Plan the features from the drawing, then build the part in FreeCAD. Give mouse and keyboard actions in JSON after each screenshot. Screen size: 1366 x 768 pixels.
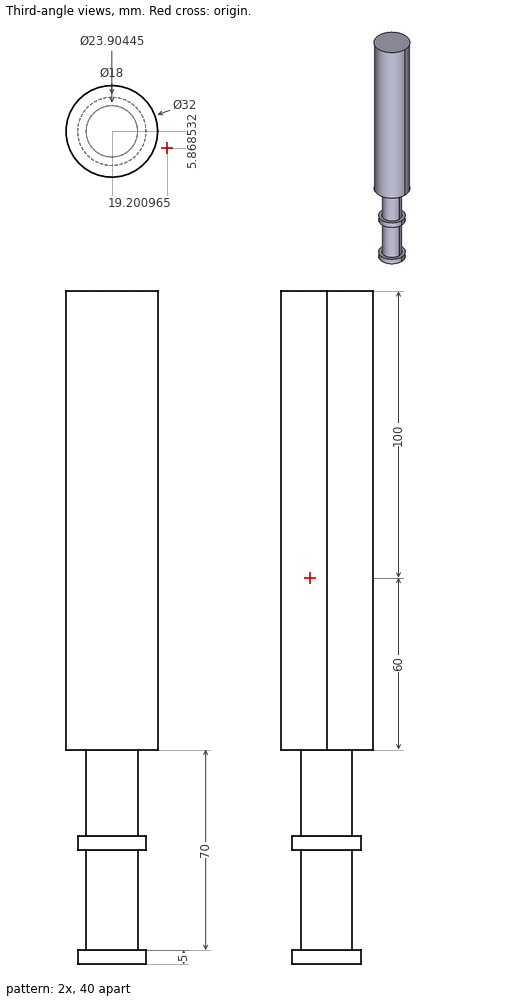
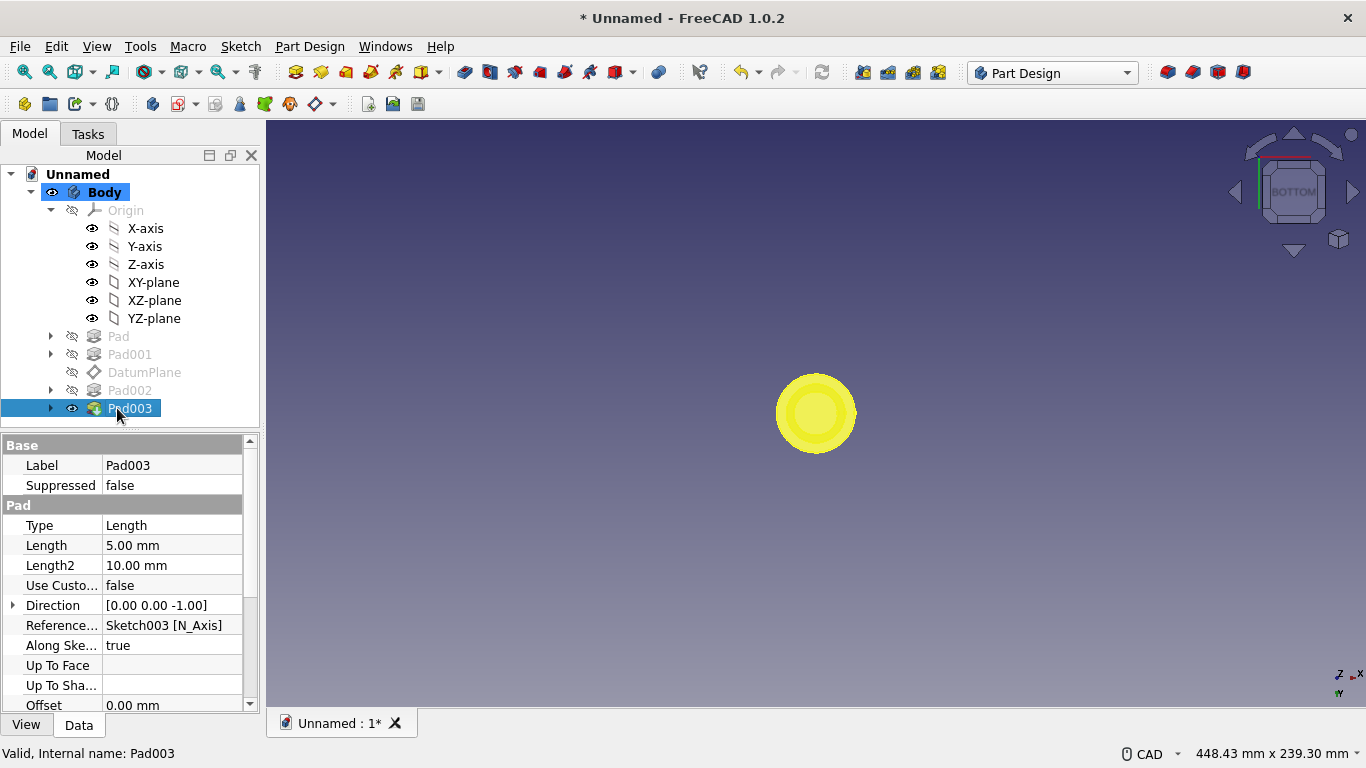
{"action": "left_click", "coordinate": [888, 72]}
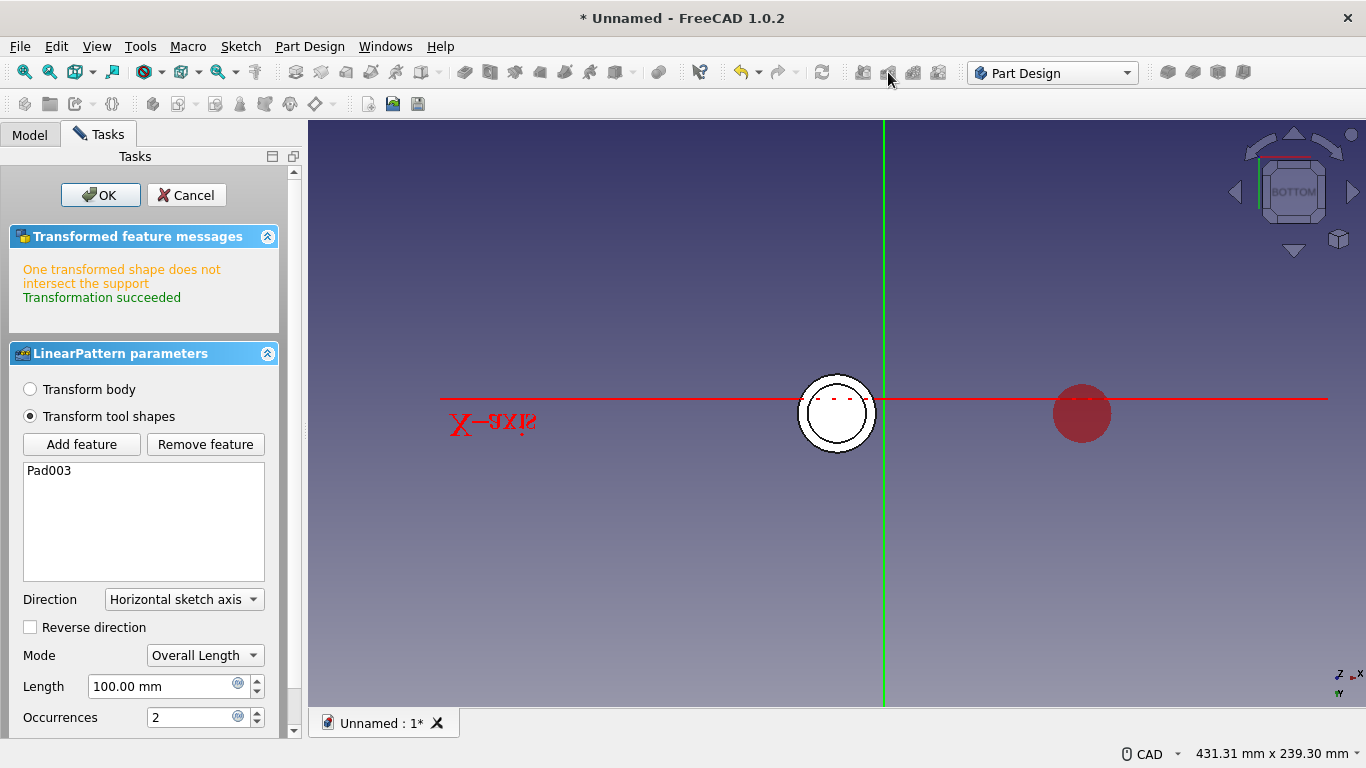
{"action": "left_click", "coordinate": [185, 600]}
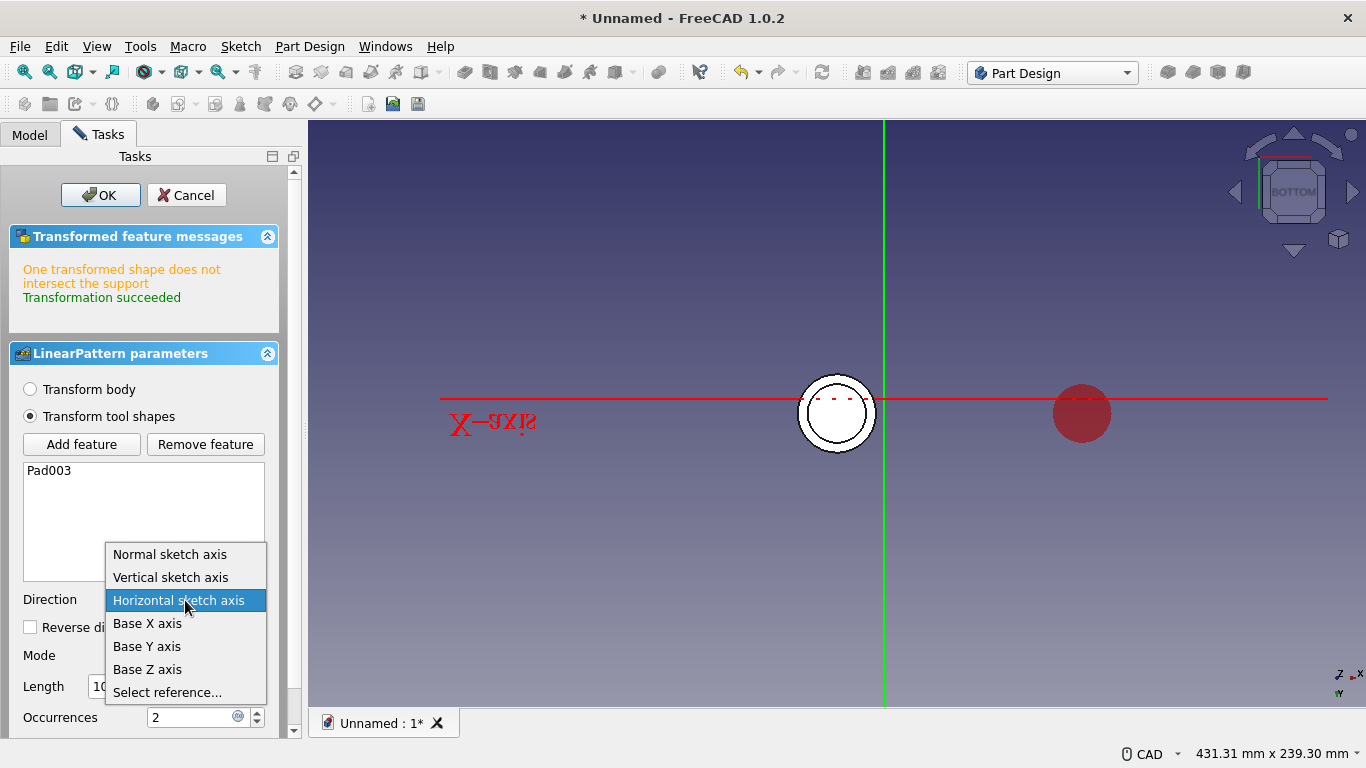
{"action": "left_click", "coordinate": [184, 670]}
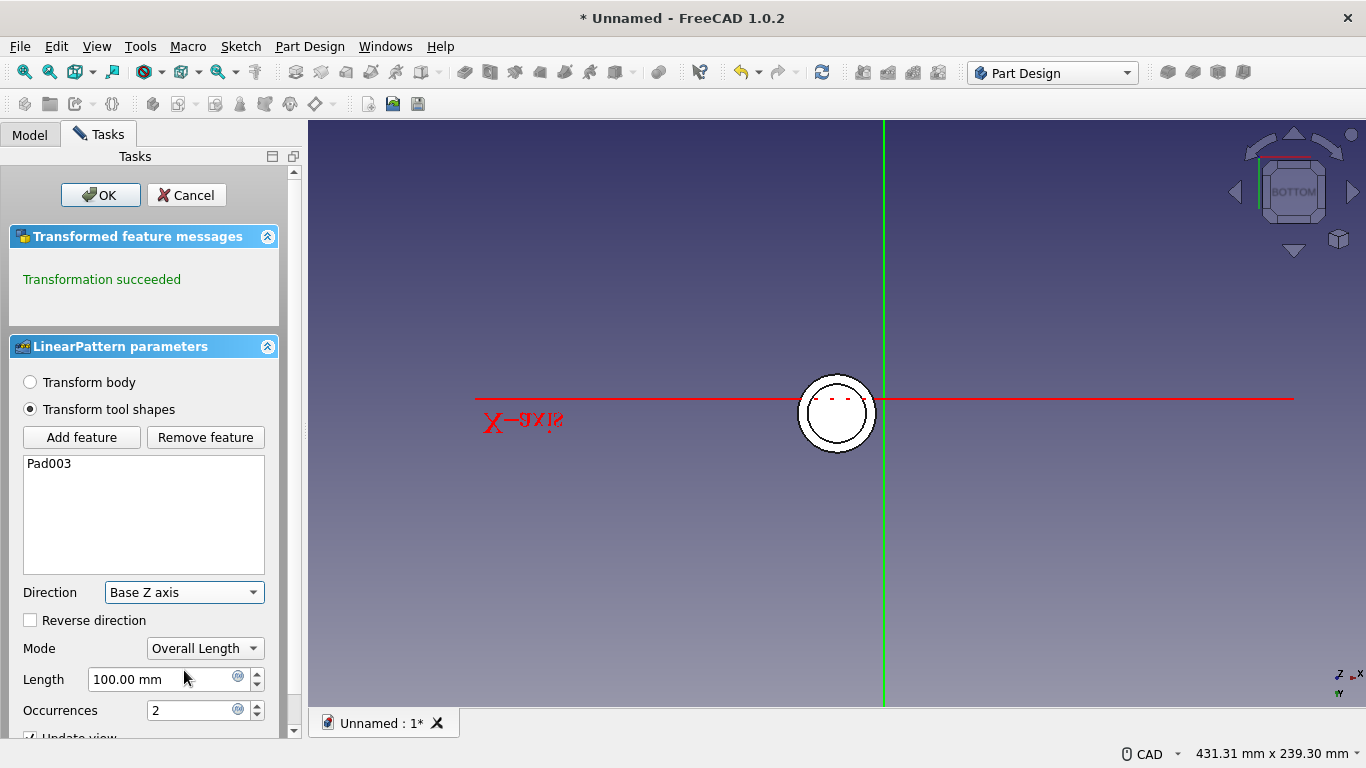
{"action": "left_click", "coordinate": [206, 648]}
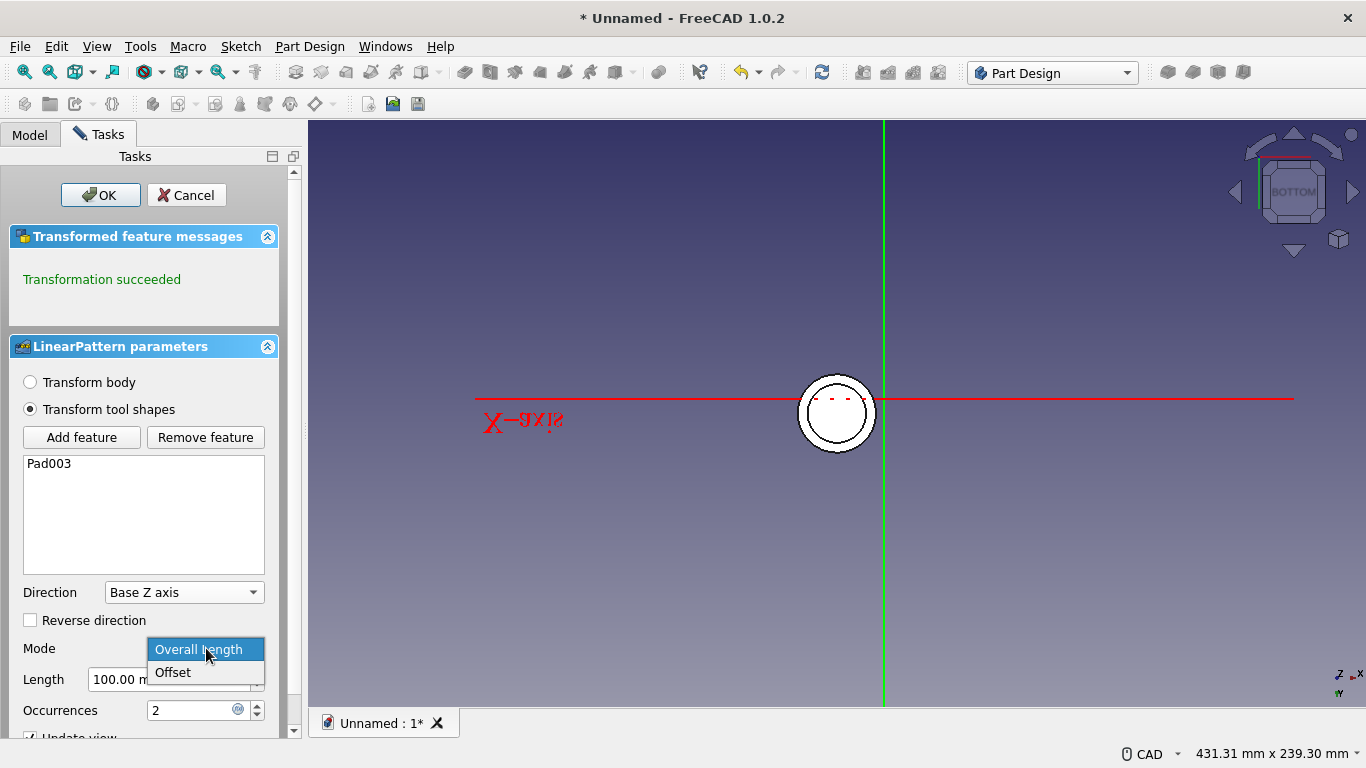
{"action": "left_click", "coordinate": [204, 672]}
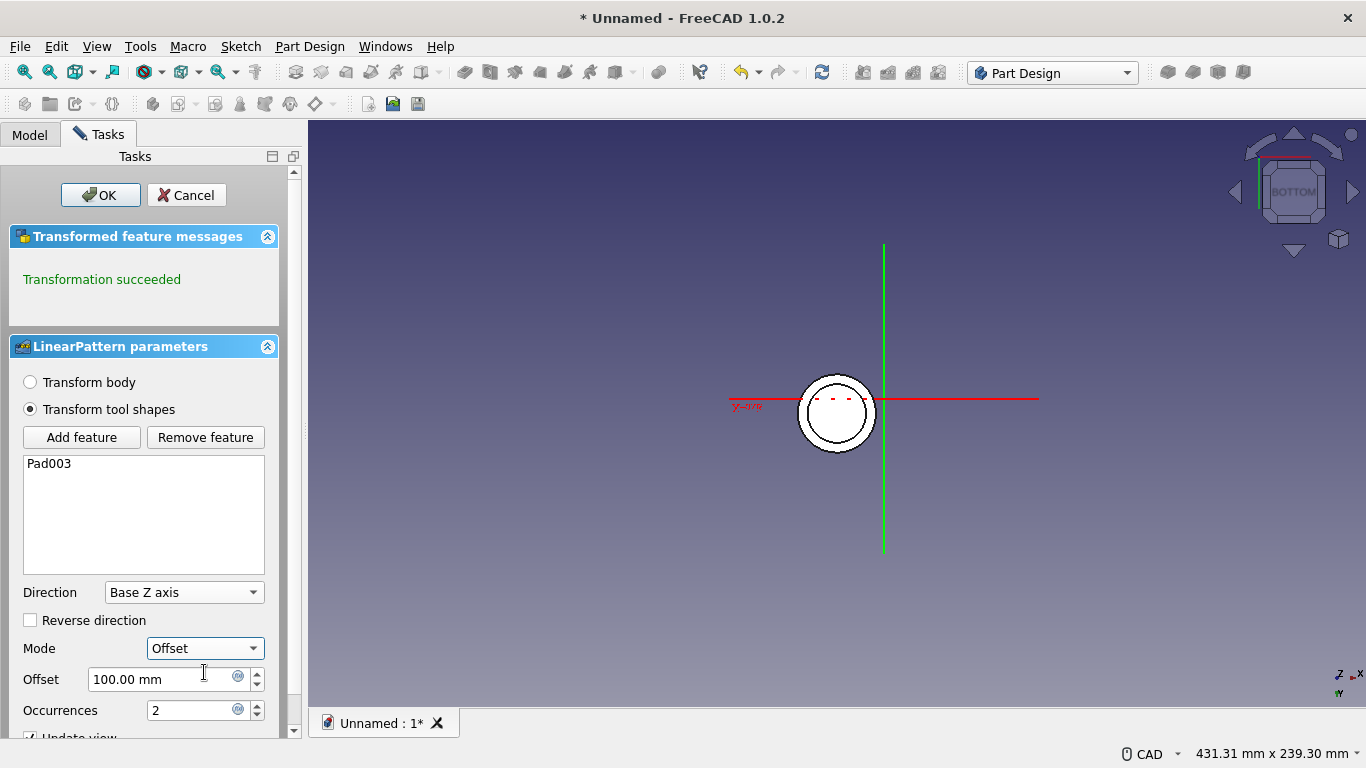
{"action": "triple_click", "coordinate": [170, 680]}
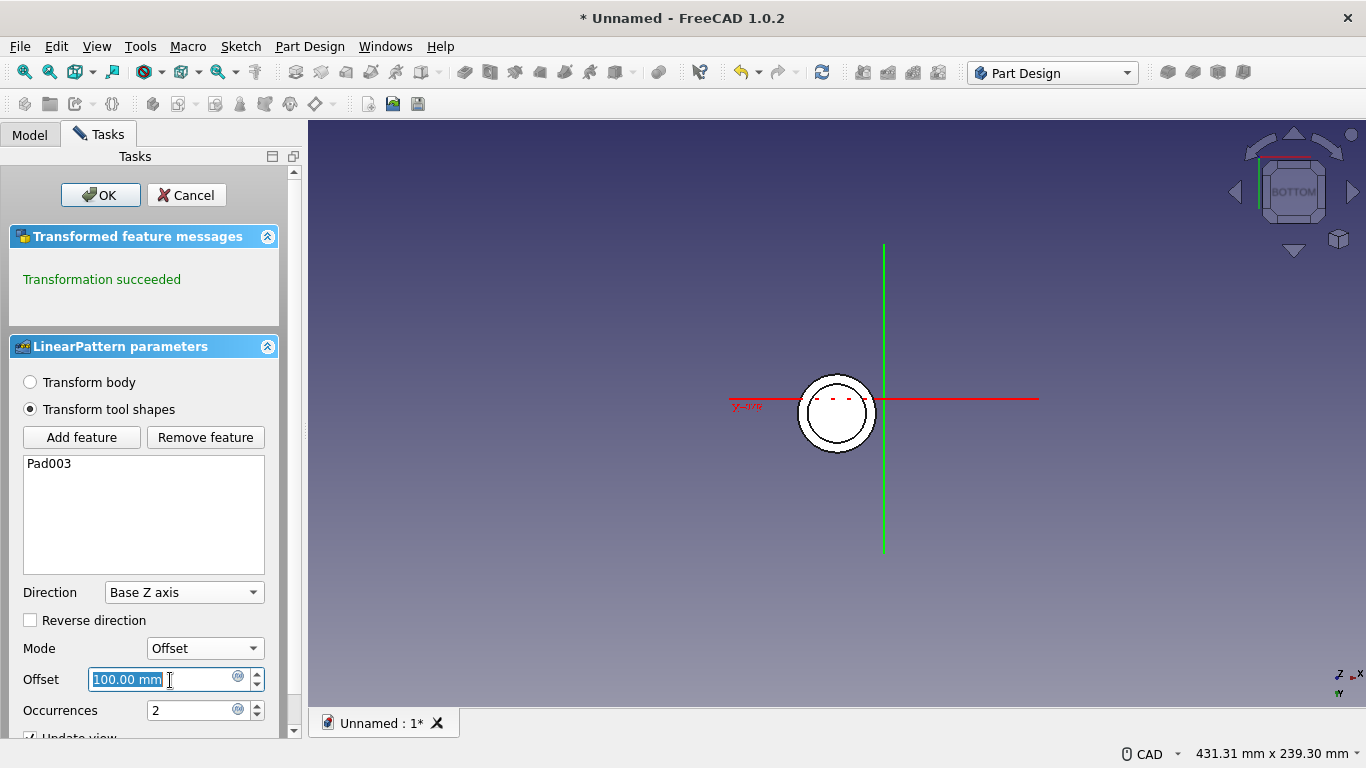
{"action": "type", "text": "40"}
{"action": "key", "text": "Tab"}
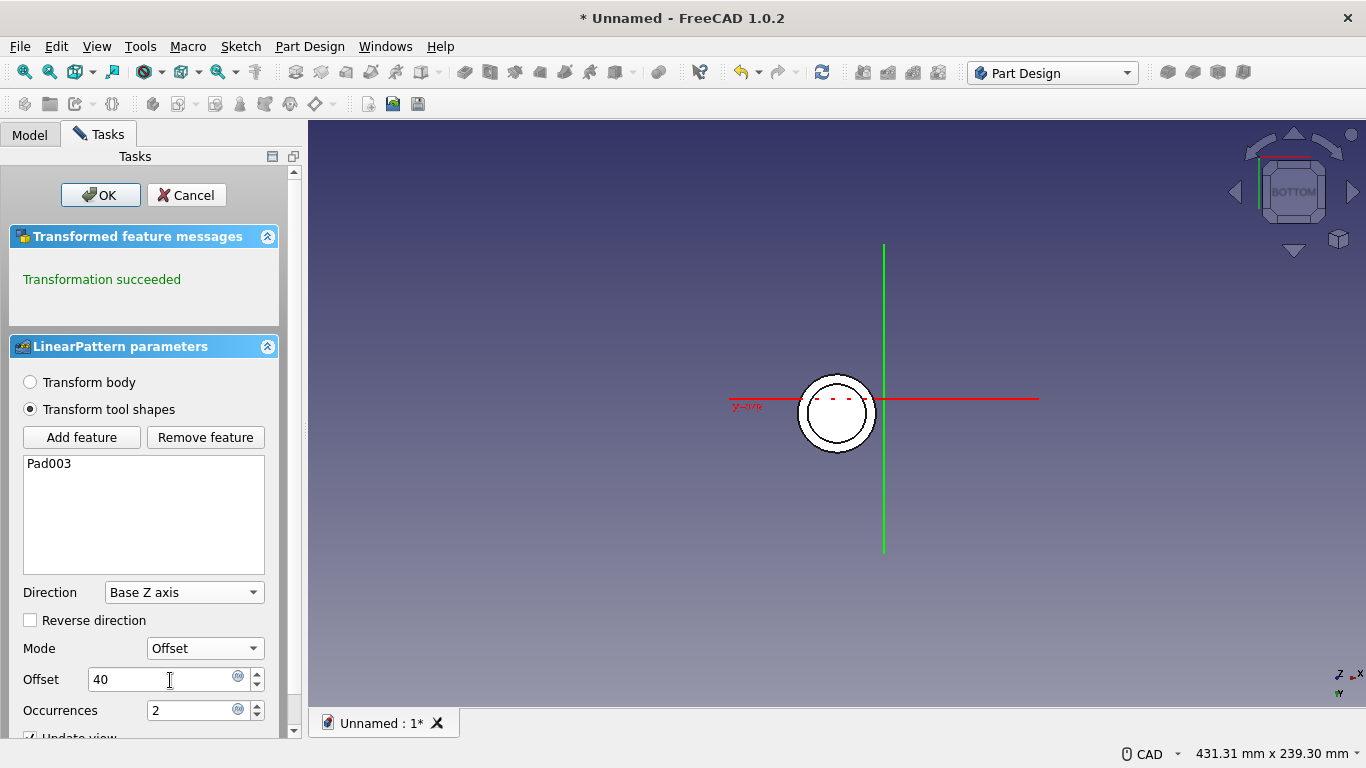
{"action": "triple_click", "coordinate": [199, 710]}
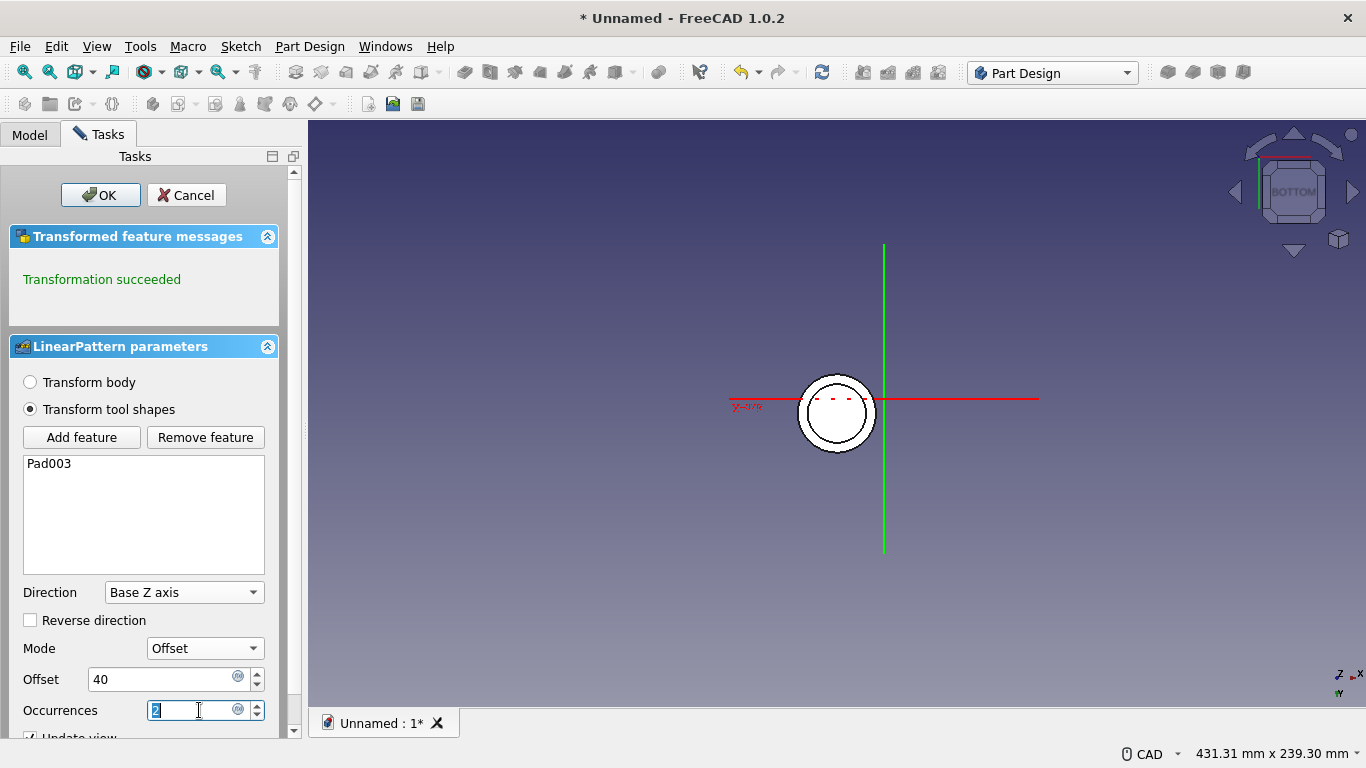
{"action": "type", "text": "2"}
{"action": "key", "text": "Tab"}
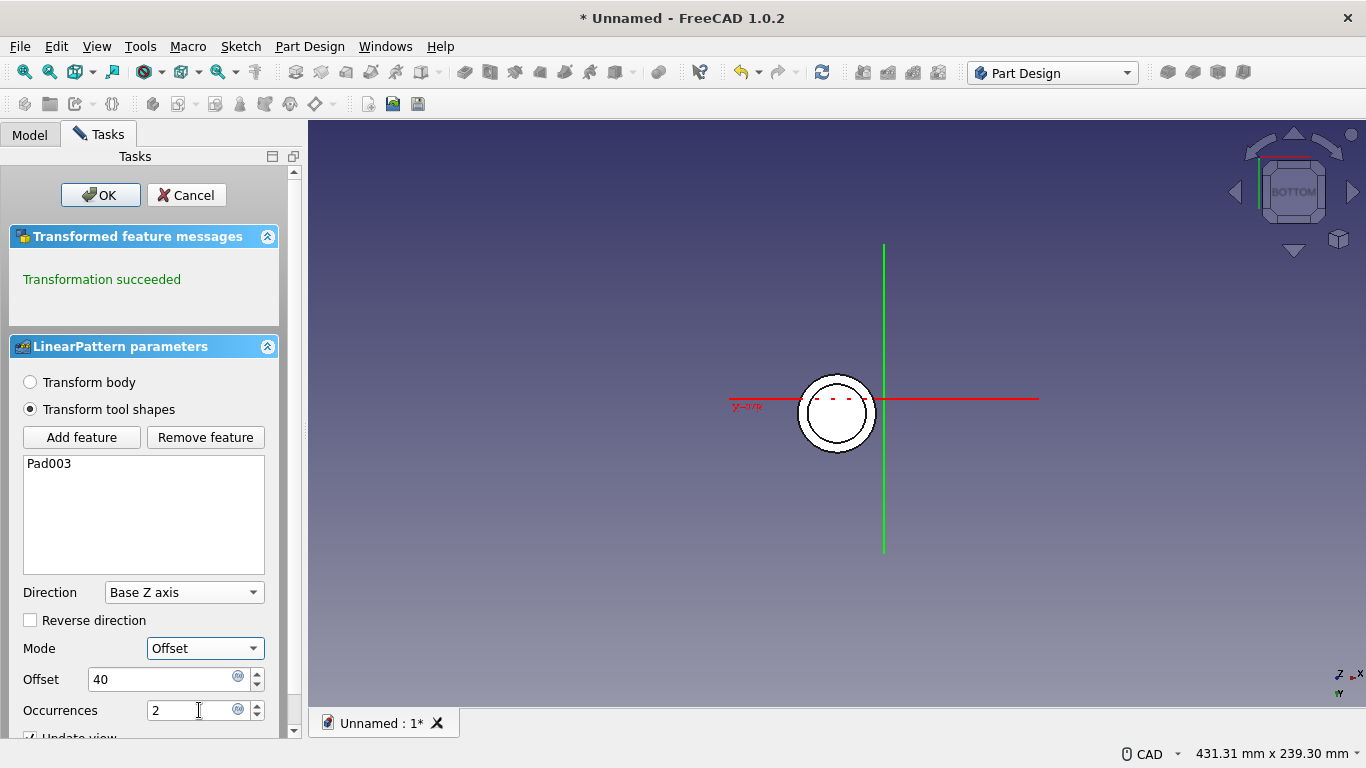
{"action": "left_click", "coordinate": [101, 195]}